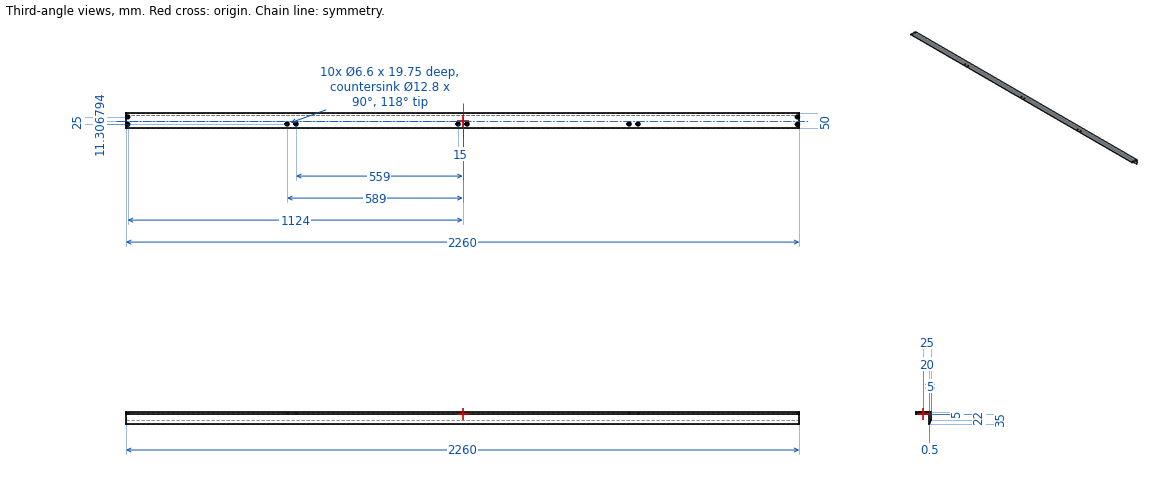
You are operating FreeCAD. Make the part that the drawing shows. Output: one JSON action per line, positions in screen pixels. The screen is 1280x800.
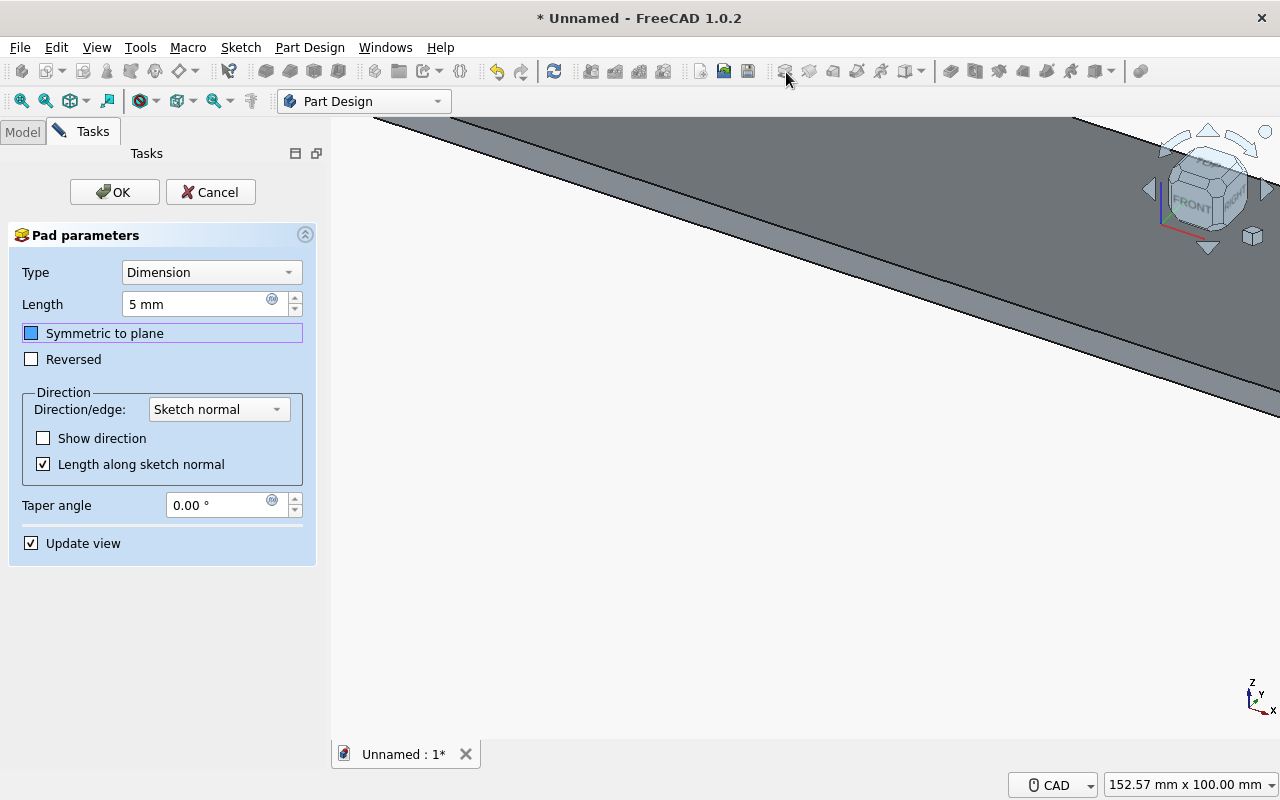
{"action": "left_click", "coordinate": [115, 192]}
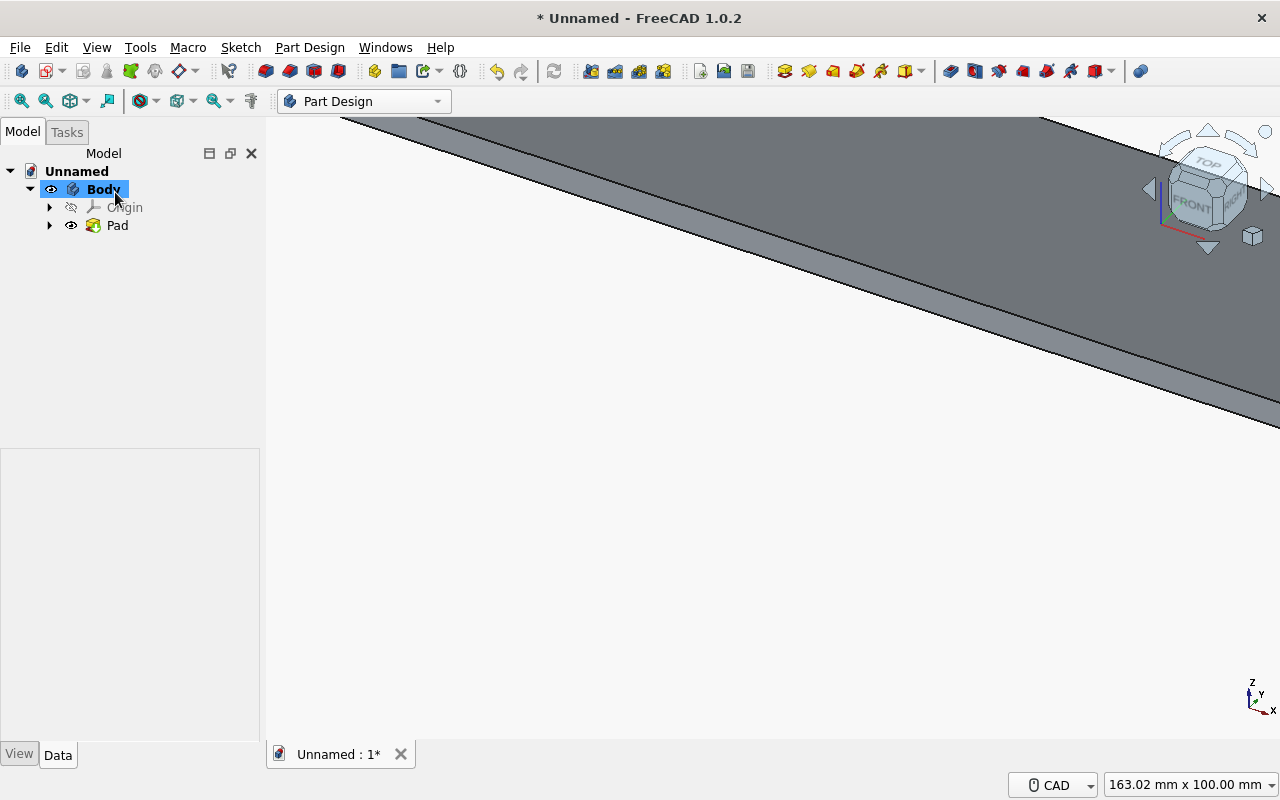
{"action": "left_click", "coordinate": [22, 102]}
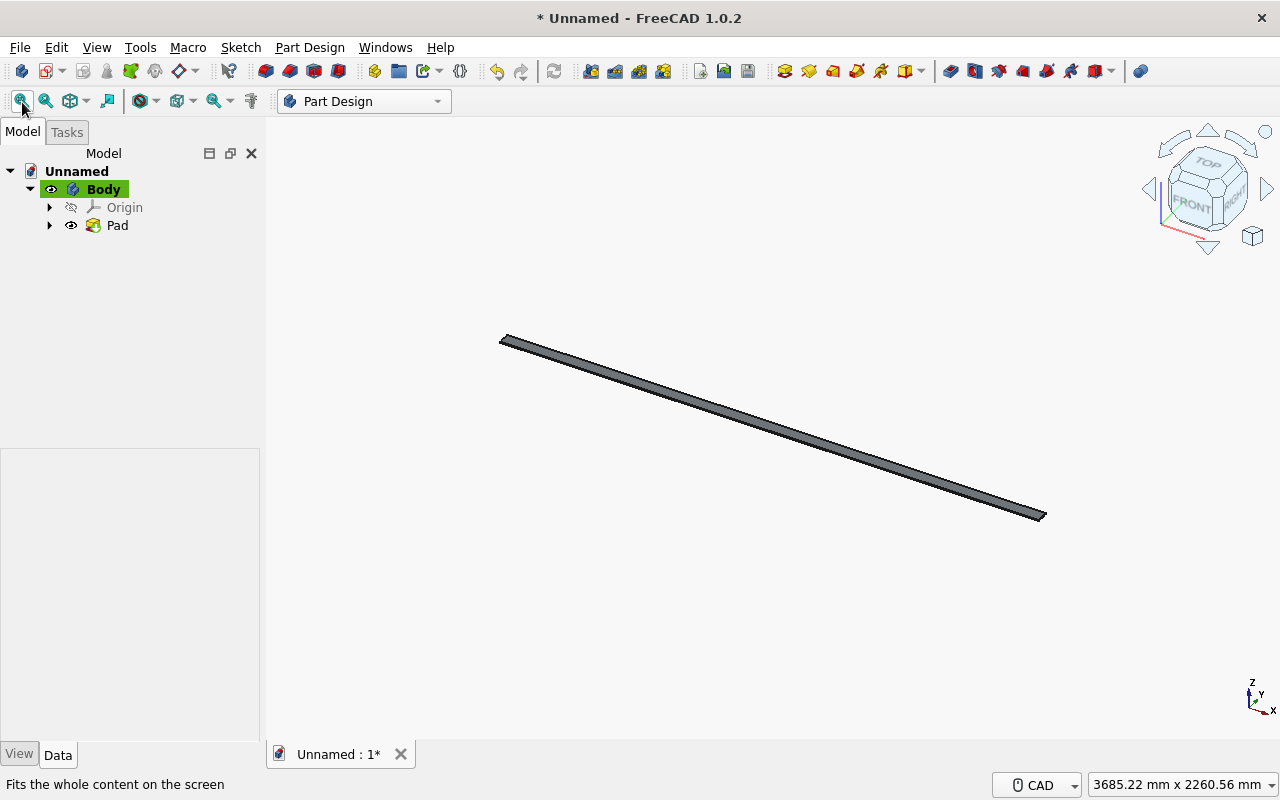
{"action": "key", "text": "6"}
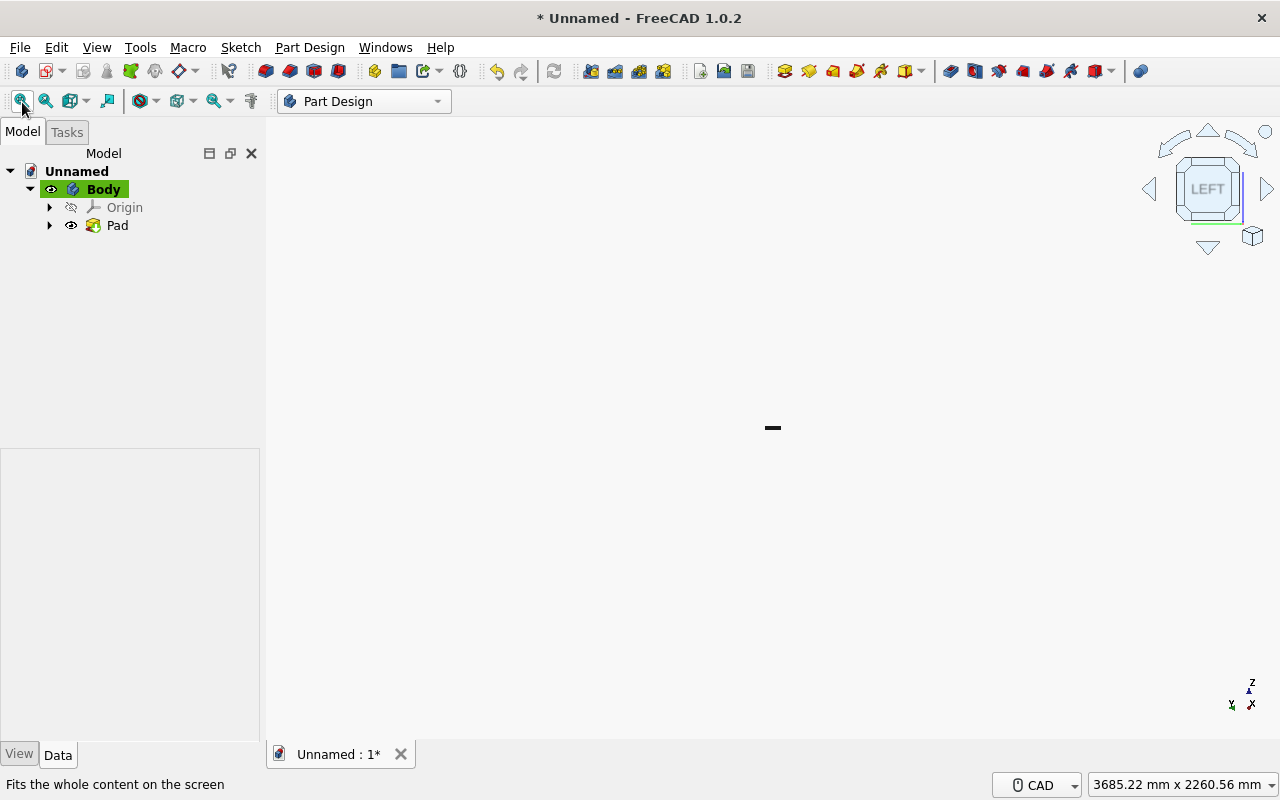
{"action": "left_click", "coordinate": [22, 102]}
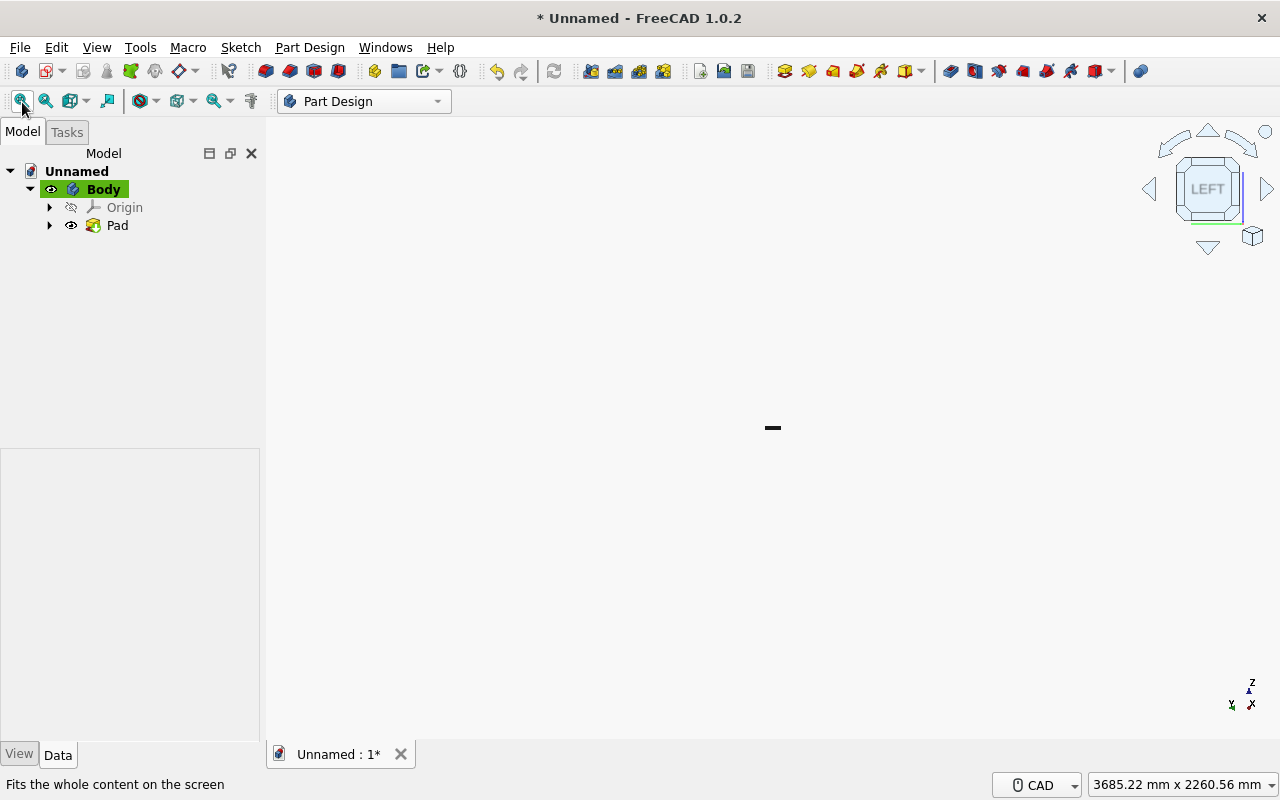
{"action": "scroll", "coordinate": [767, 427], "scroll_direction": "up", "scroll_amount": 15}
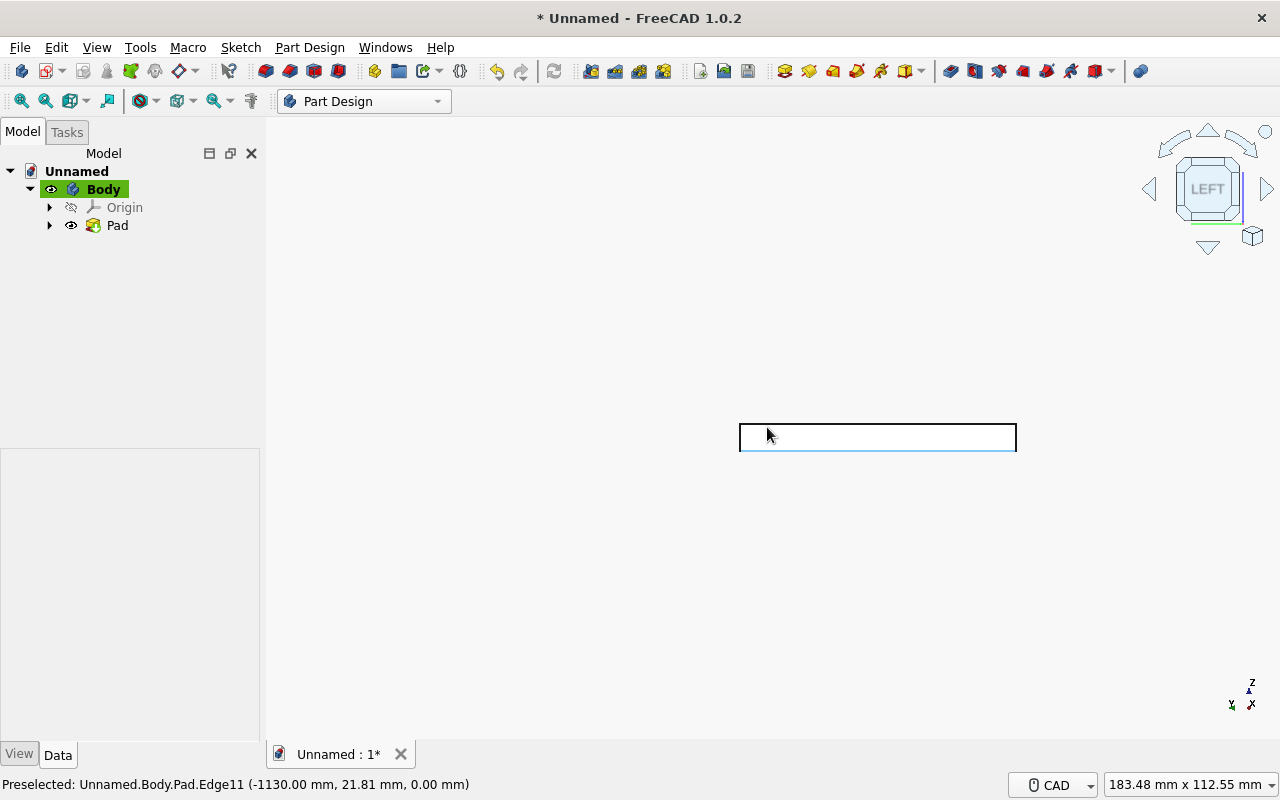
{"action": "left_click", "coordinate": [760, 437]}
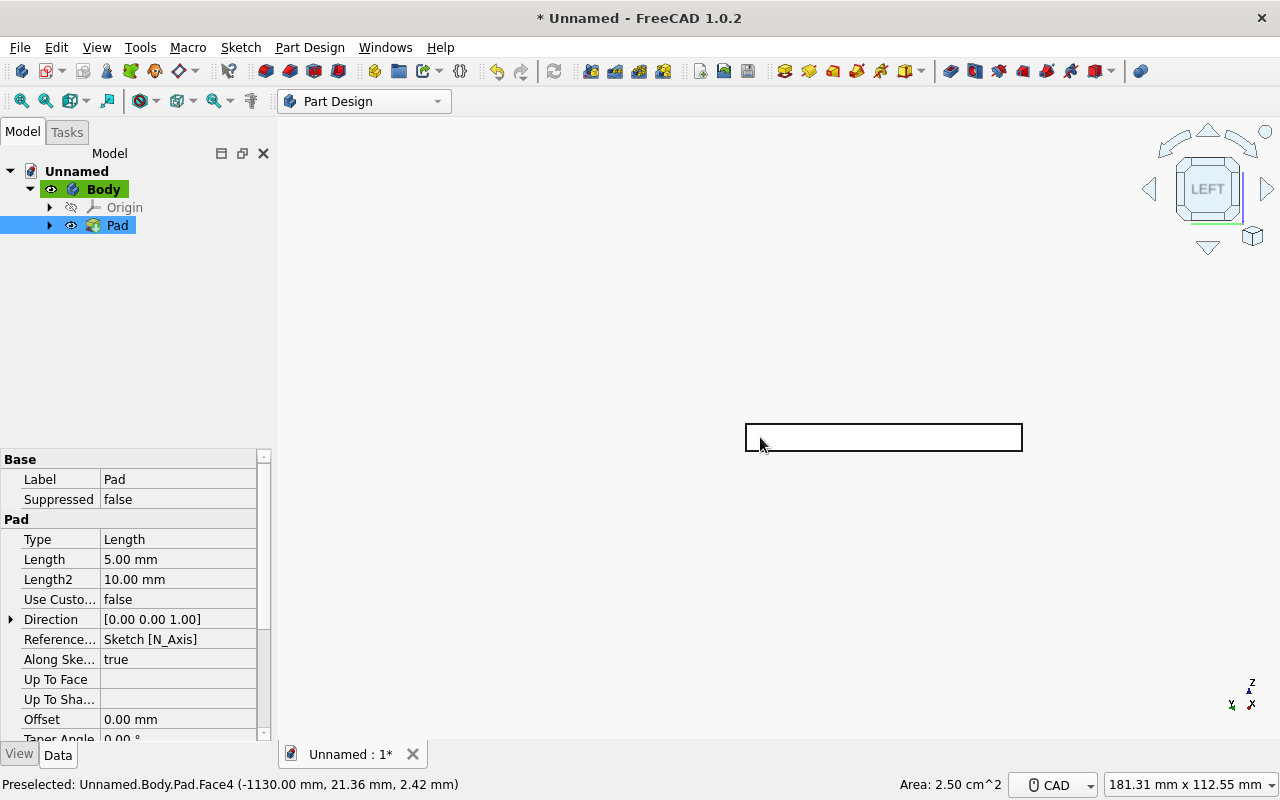
{"action": "left_click", "coordinate": [46, 72]}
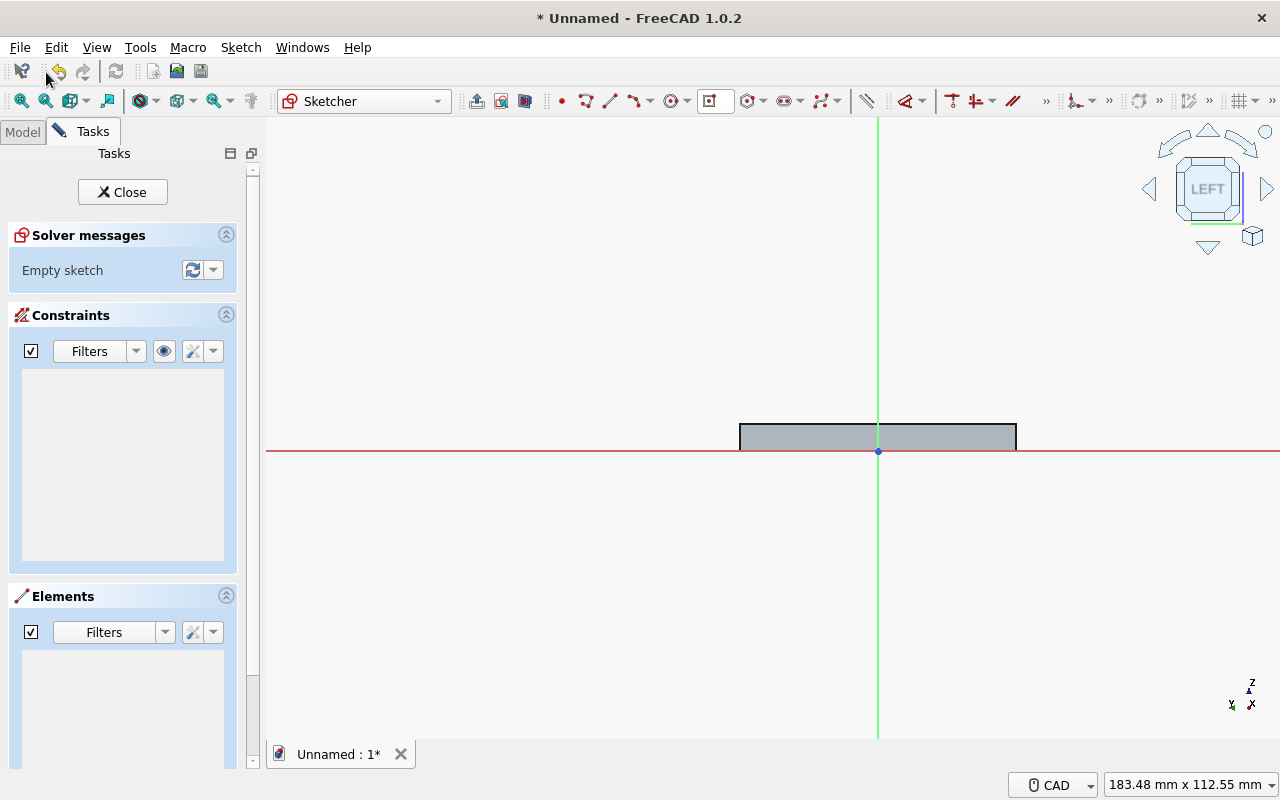
{"action": "scroll", "coordinate": [894, 646], "scroll_direction": "up", "scroll_amount": 4}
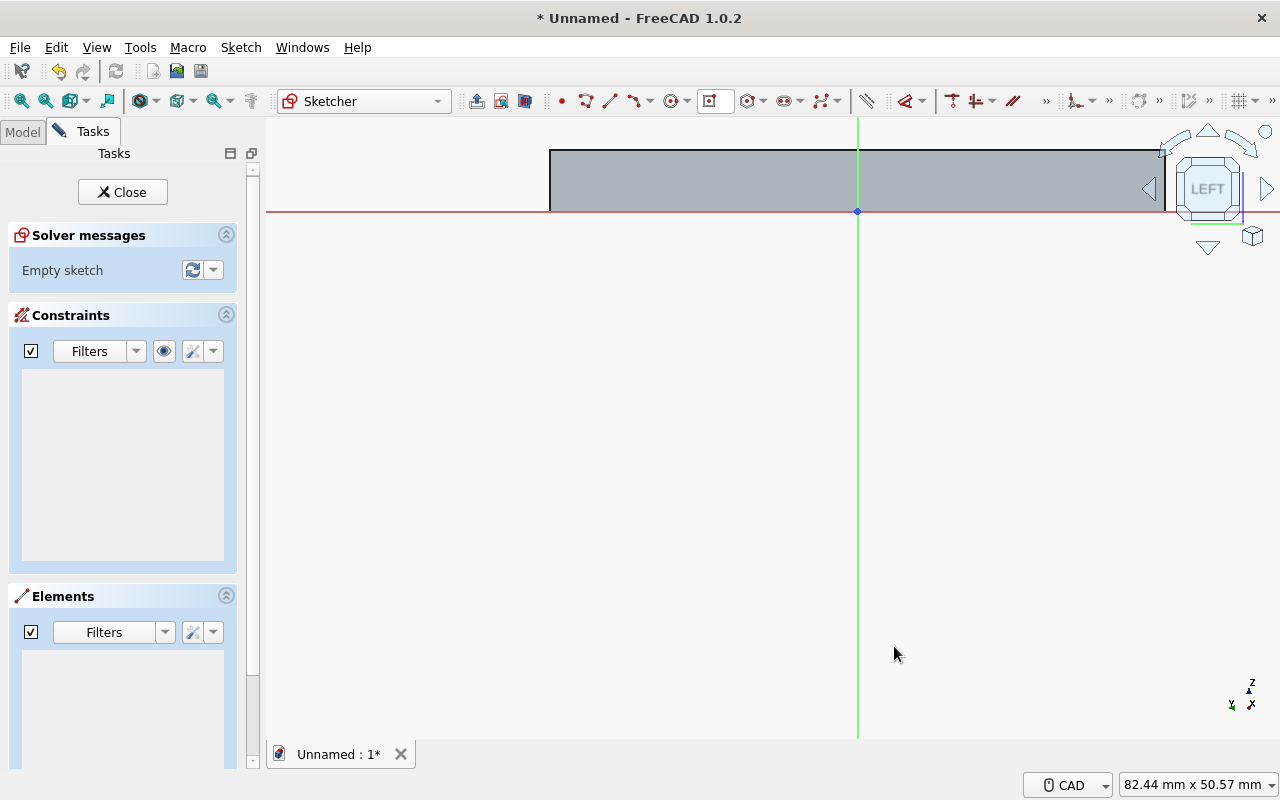
{"action": "left_click", "coordinate": [586, 102]}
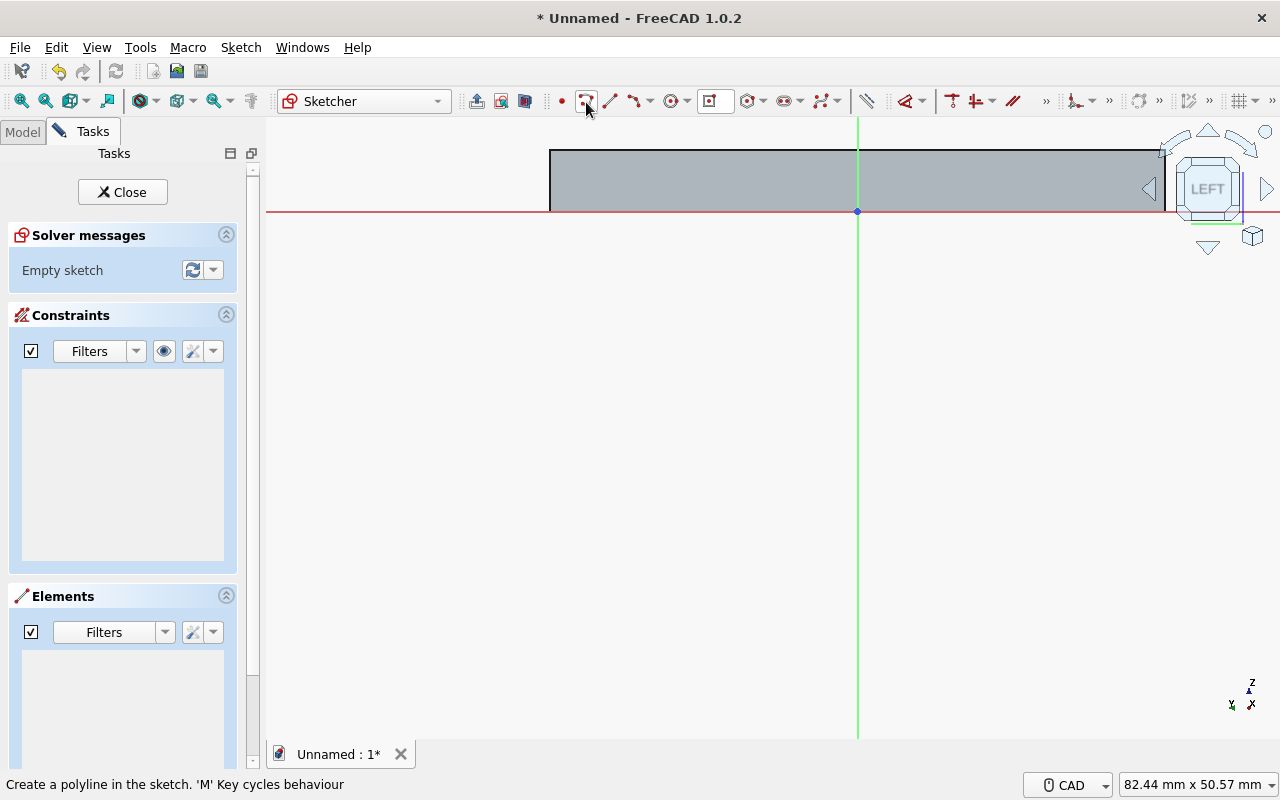
{"action": "left_click", "coordinate": [612, 212]}
{"action": "left_click", "coordinate": [550, 221]}
{"action": "left_click", "coordinate": [550, 482]}
{"action": "left_click", "coordinate": [606, 642]}